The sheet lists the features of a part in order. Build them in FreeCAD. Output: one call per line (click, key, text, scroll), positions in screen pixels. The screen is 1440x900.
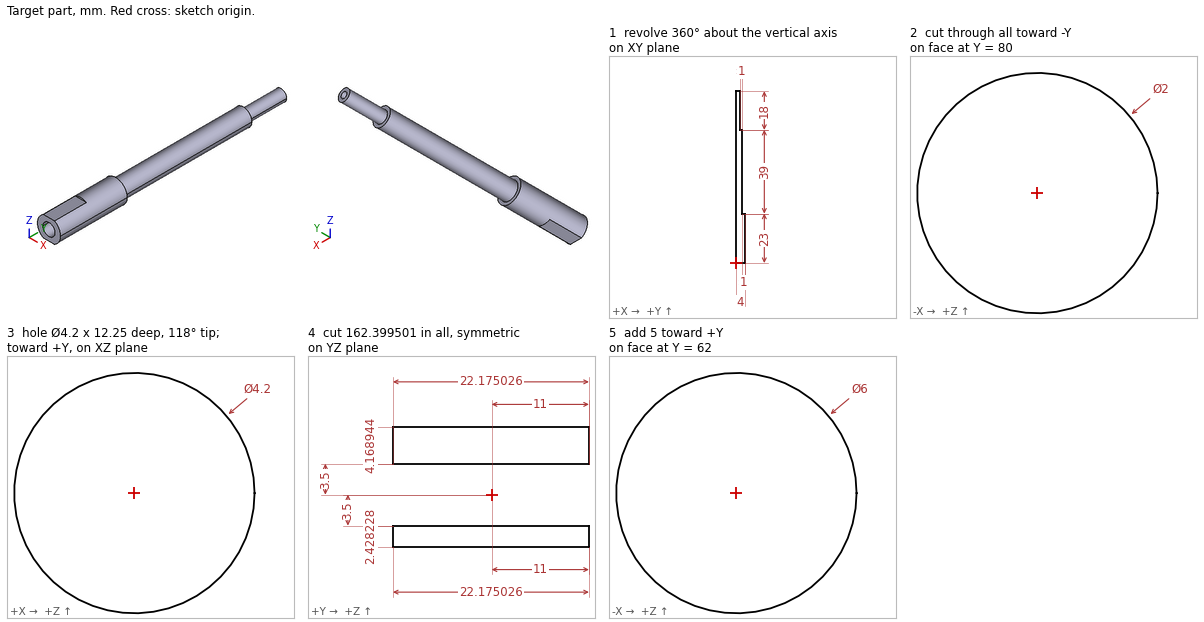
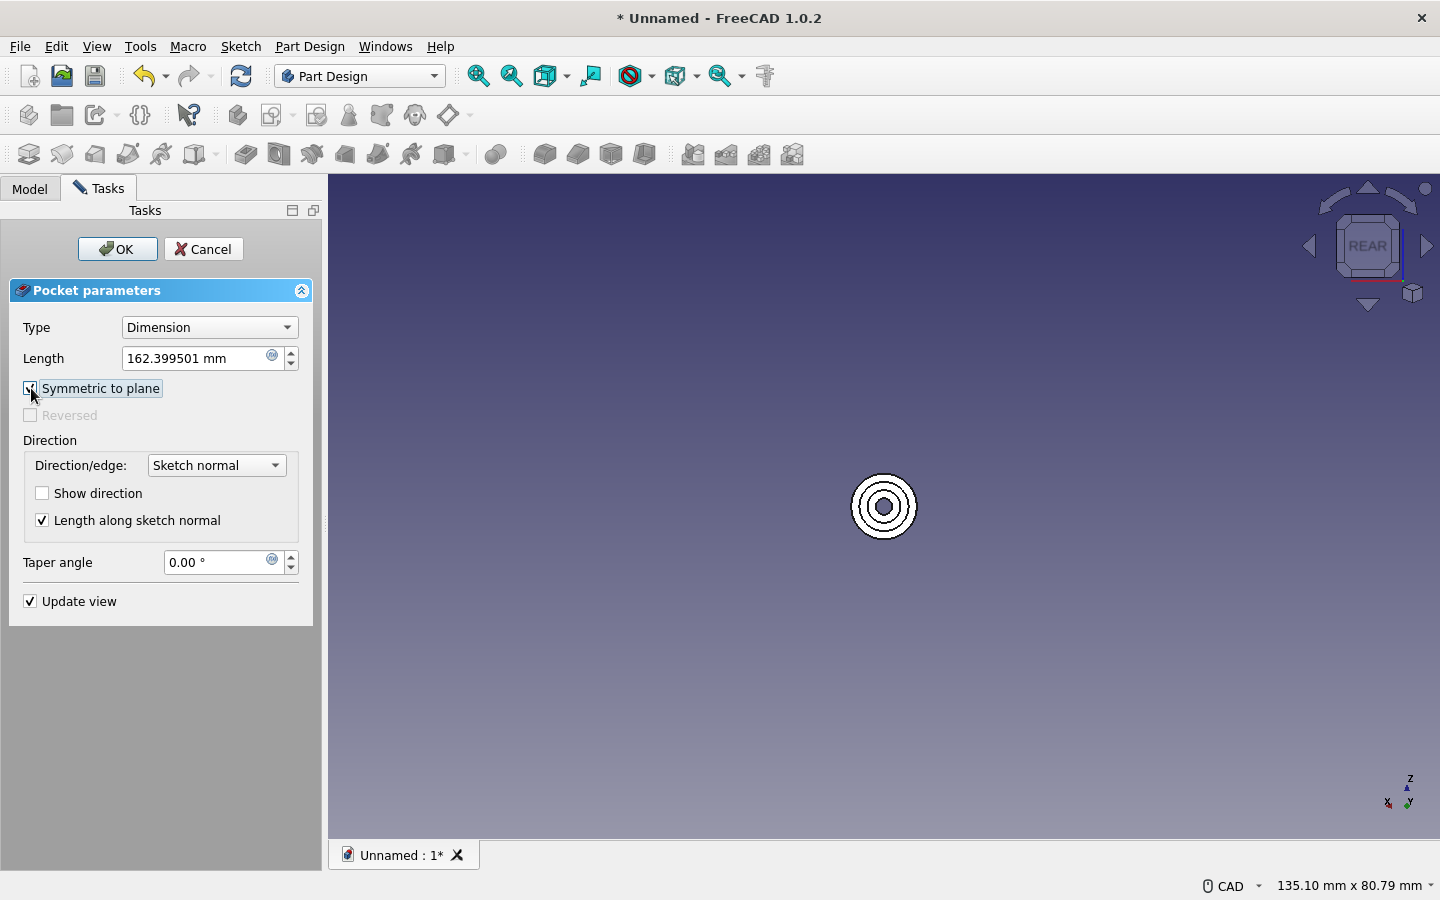
click(118, 249)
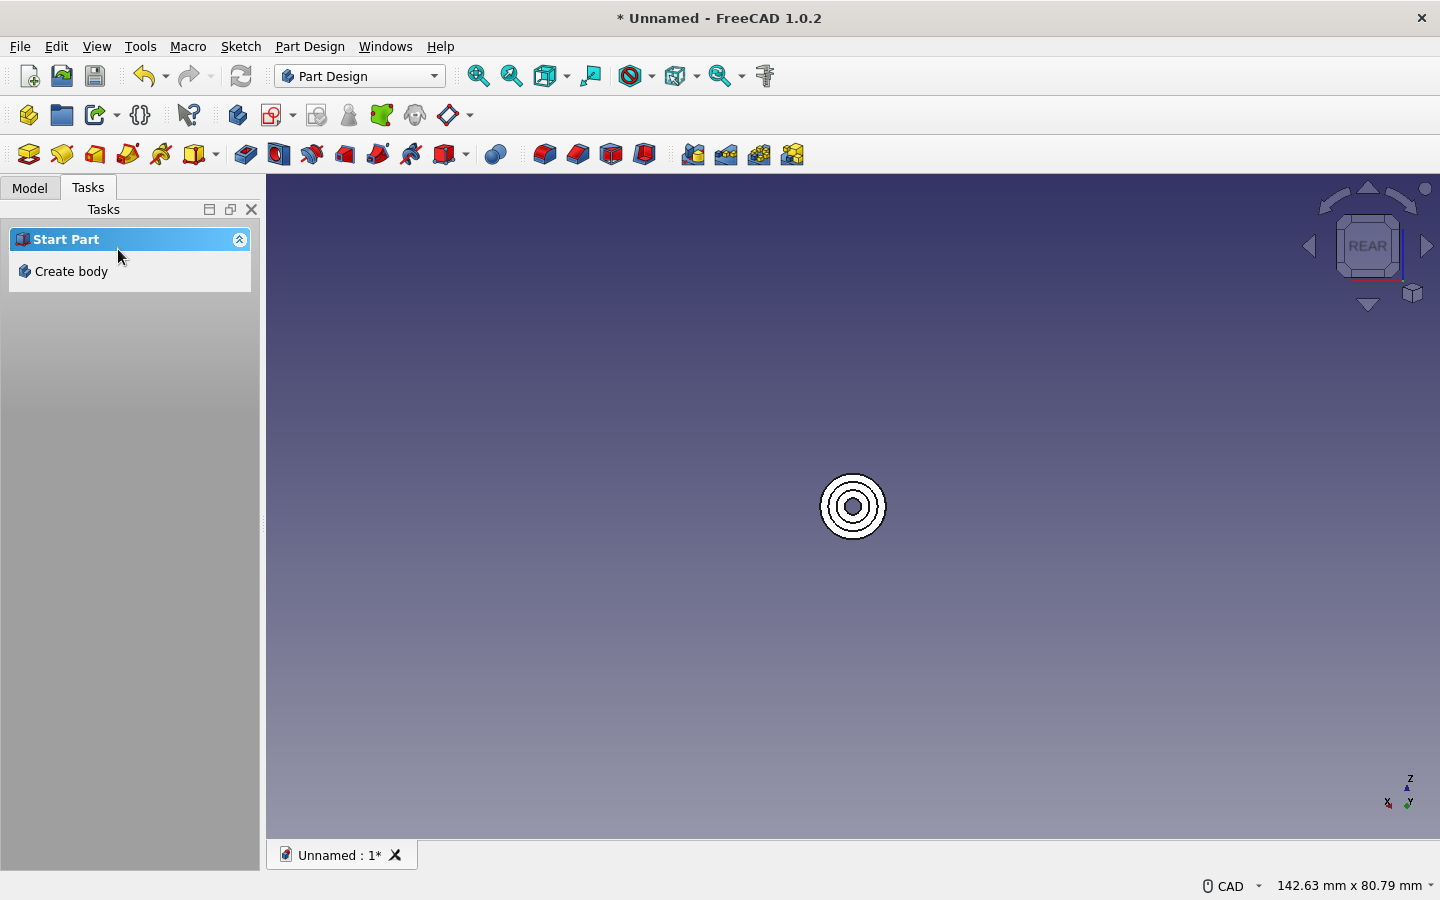
key(v)
key(f)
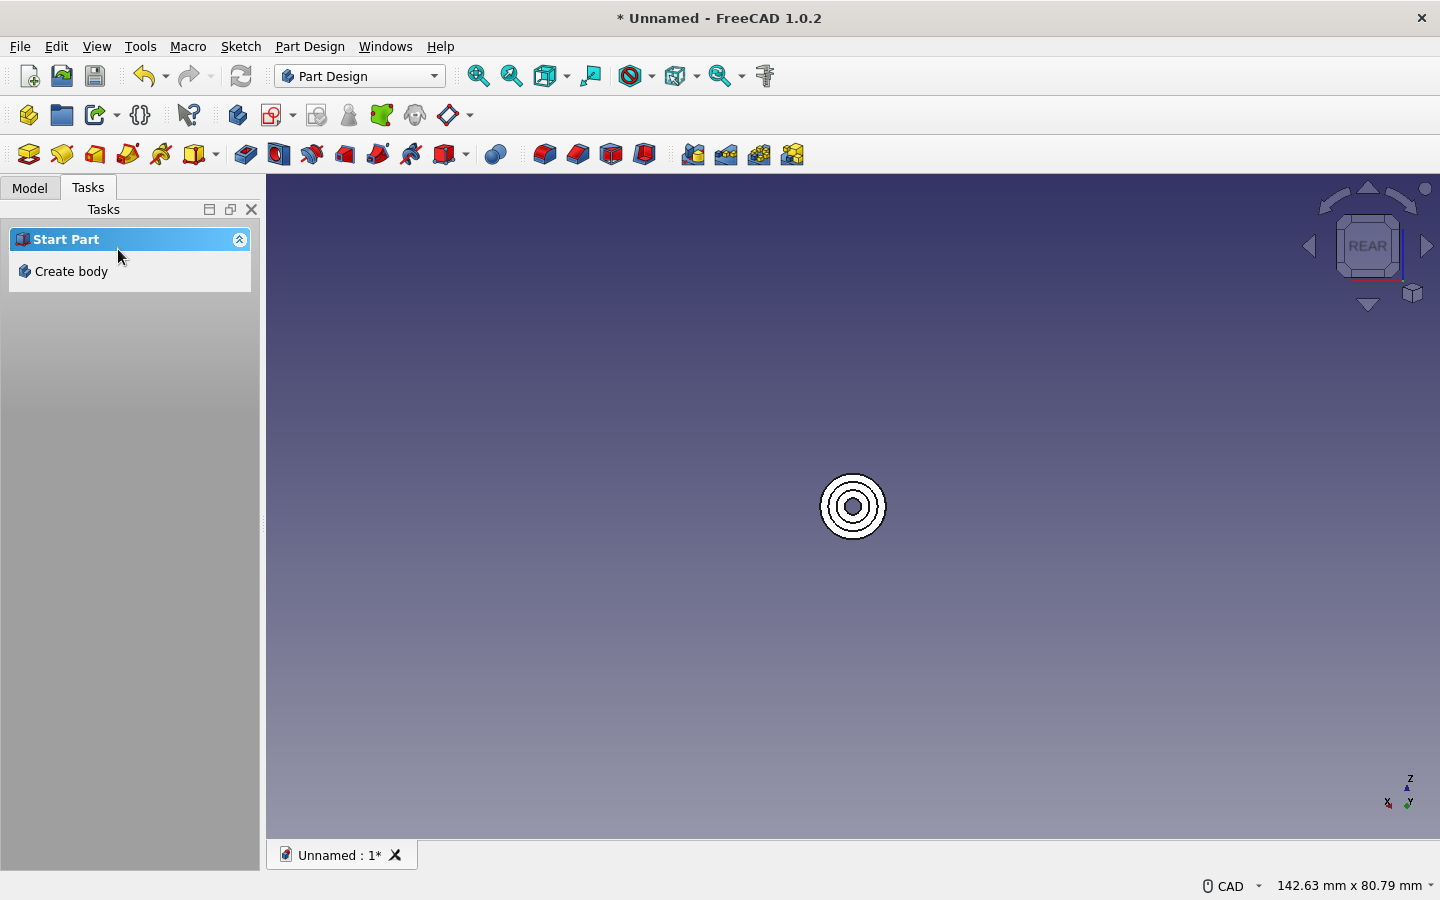
scroll(832, 505, up, 7)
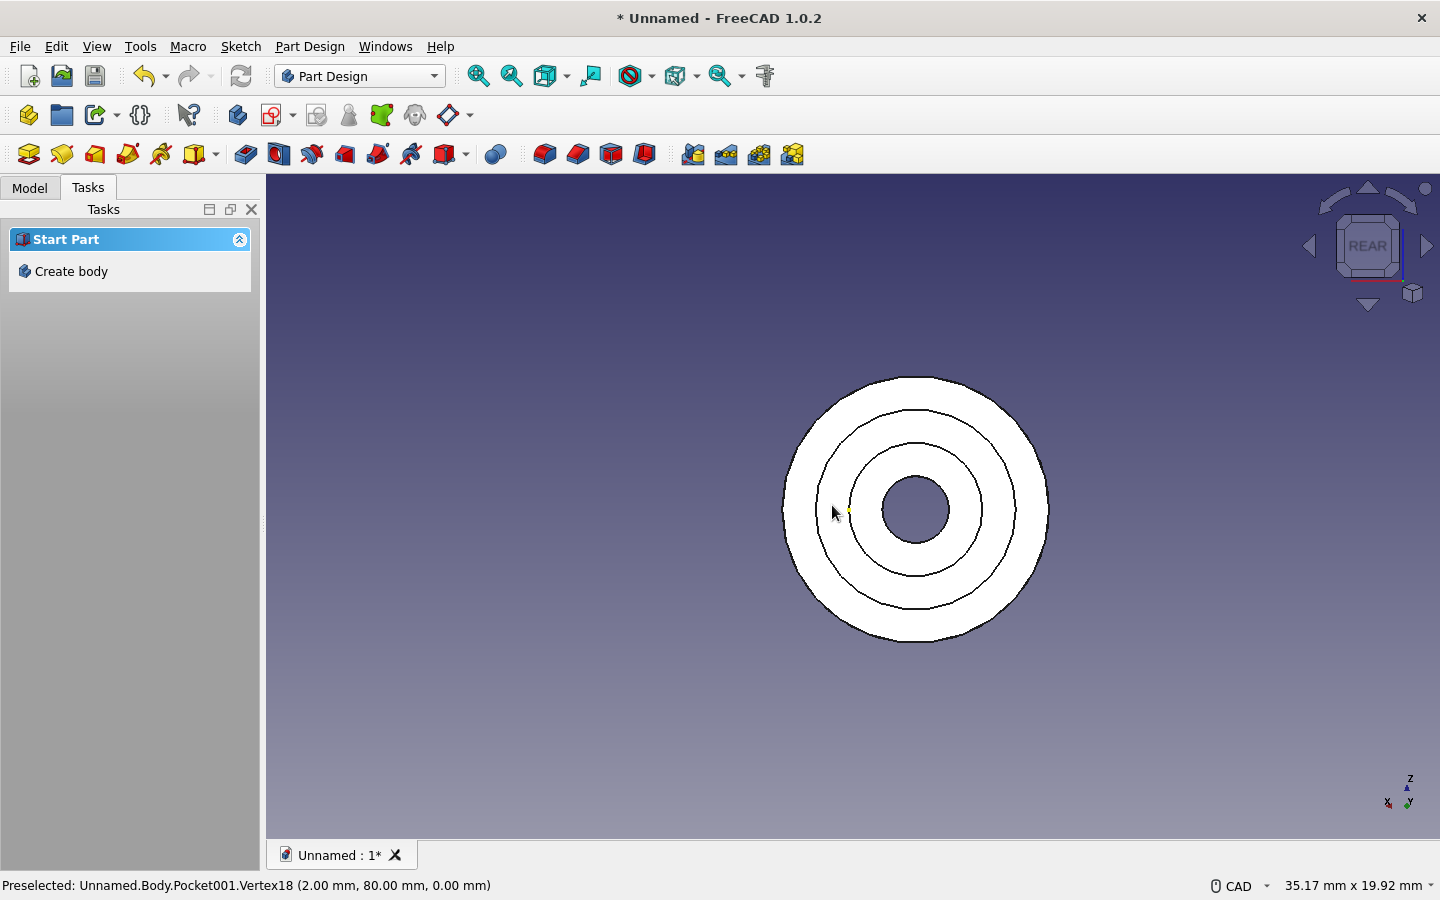
click(830, 509)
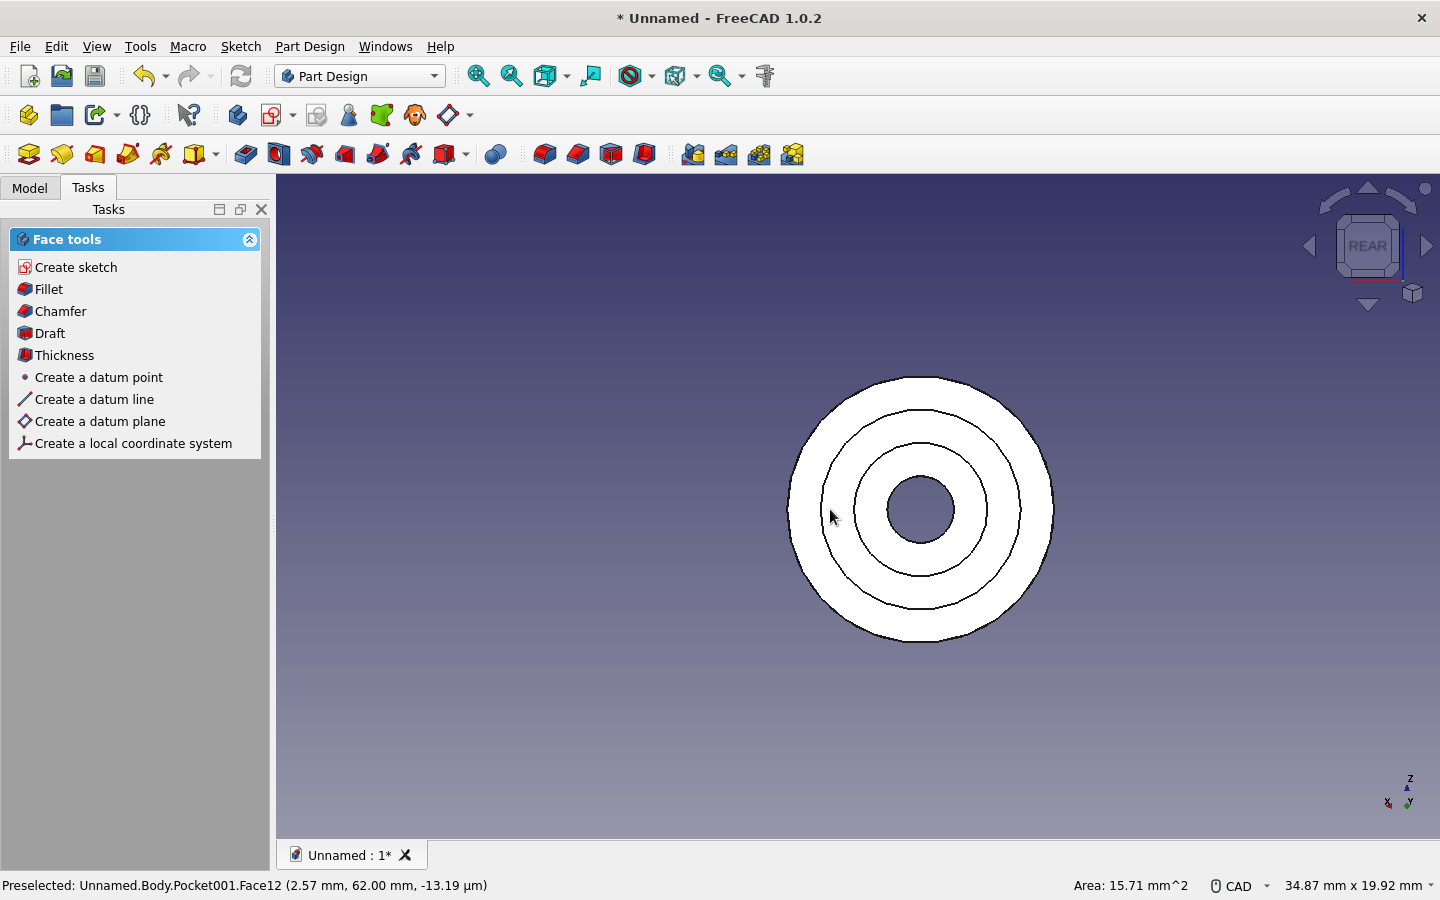
click(270, 116)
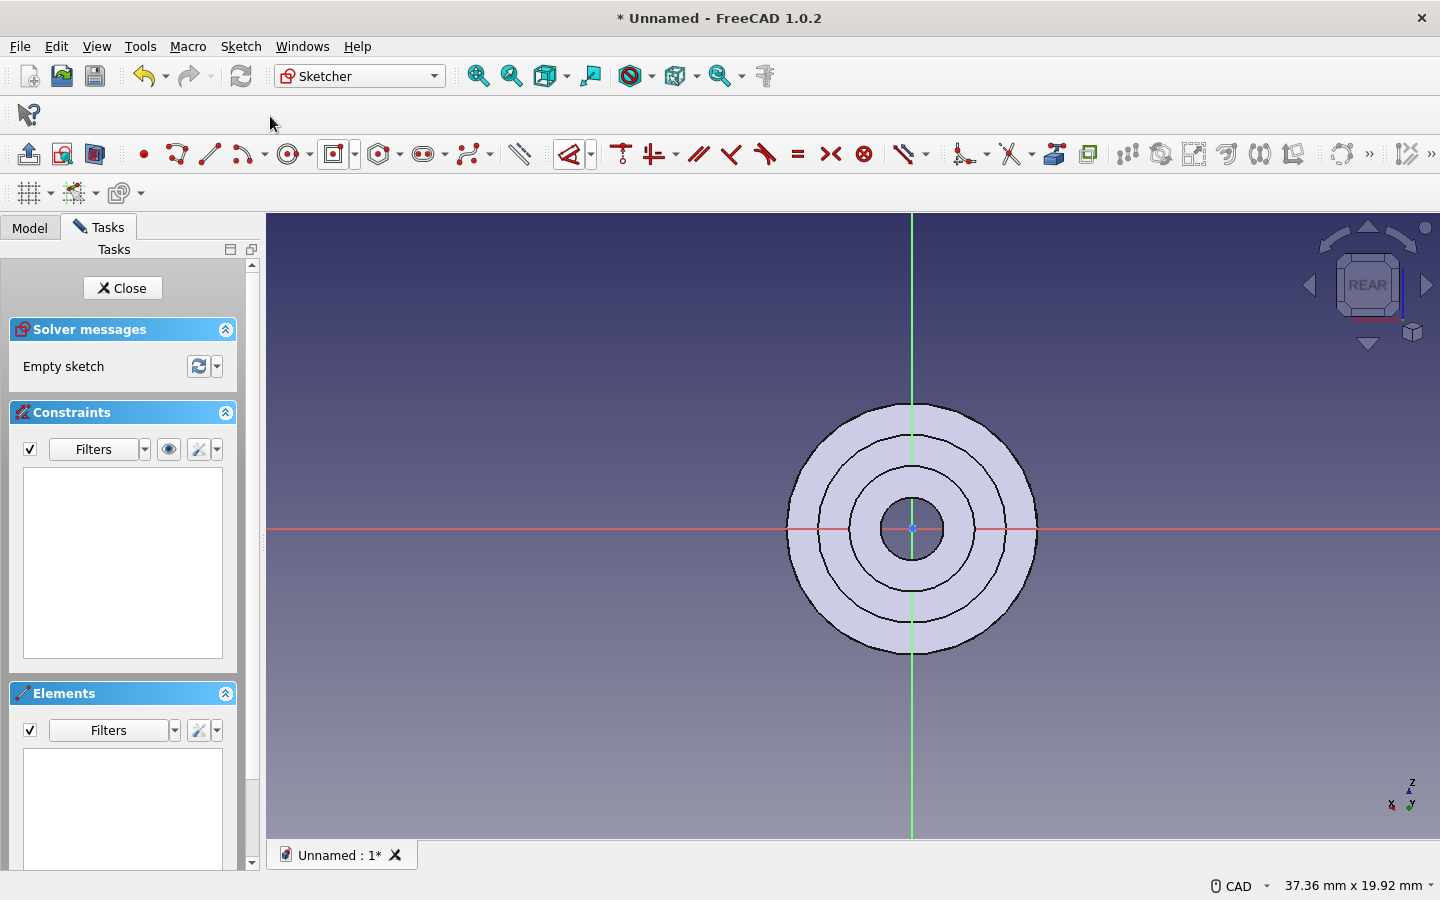
scroll(1016, 531, up, 4)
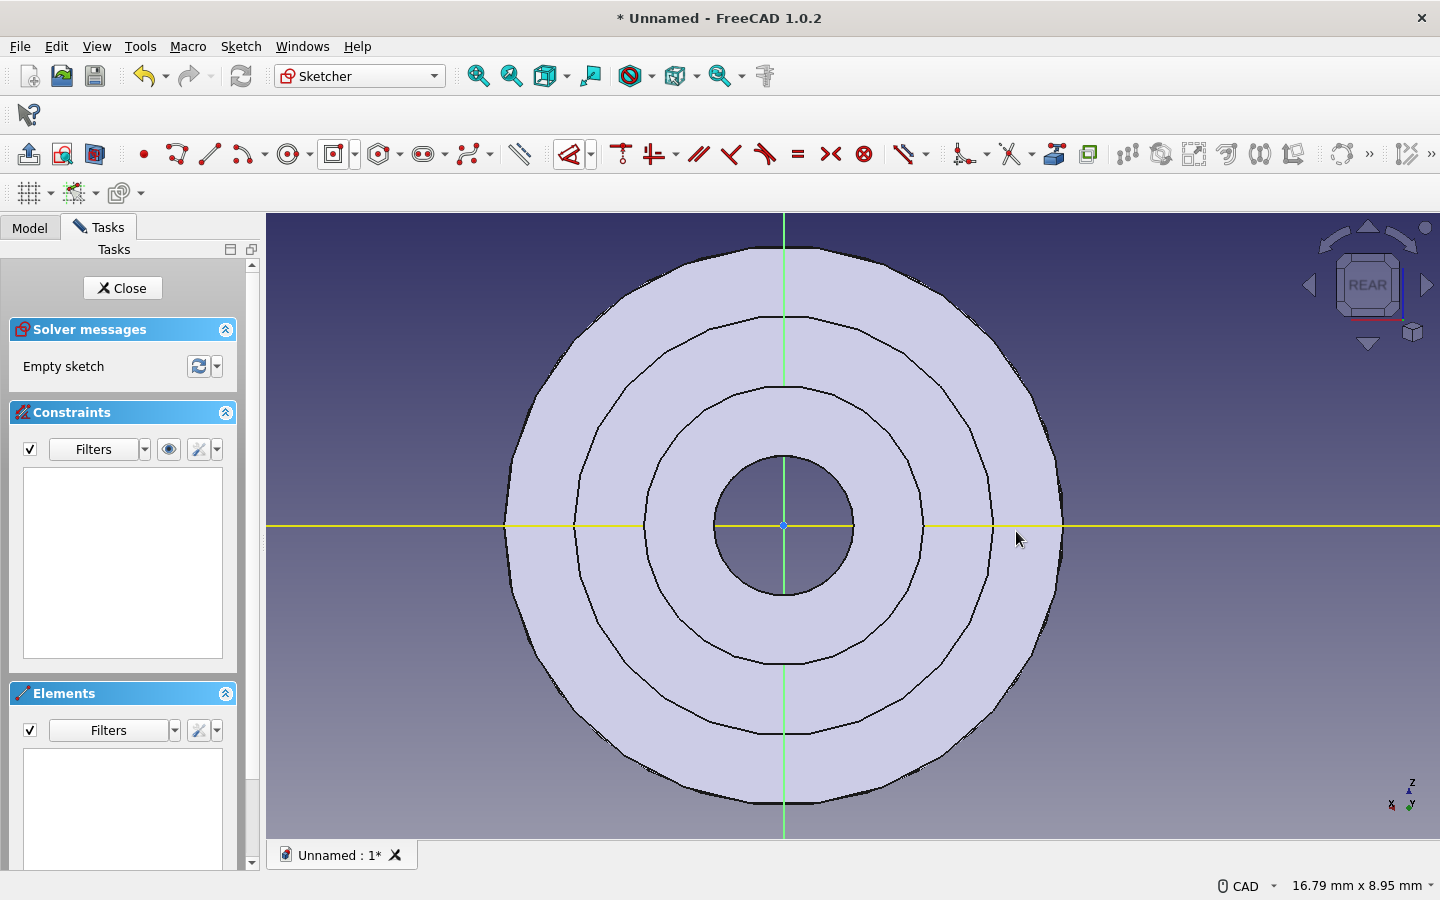
click(288, 154)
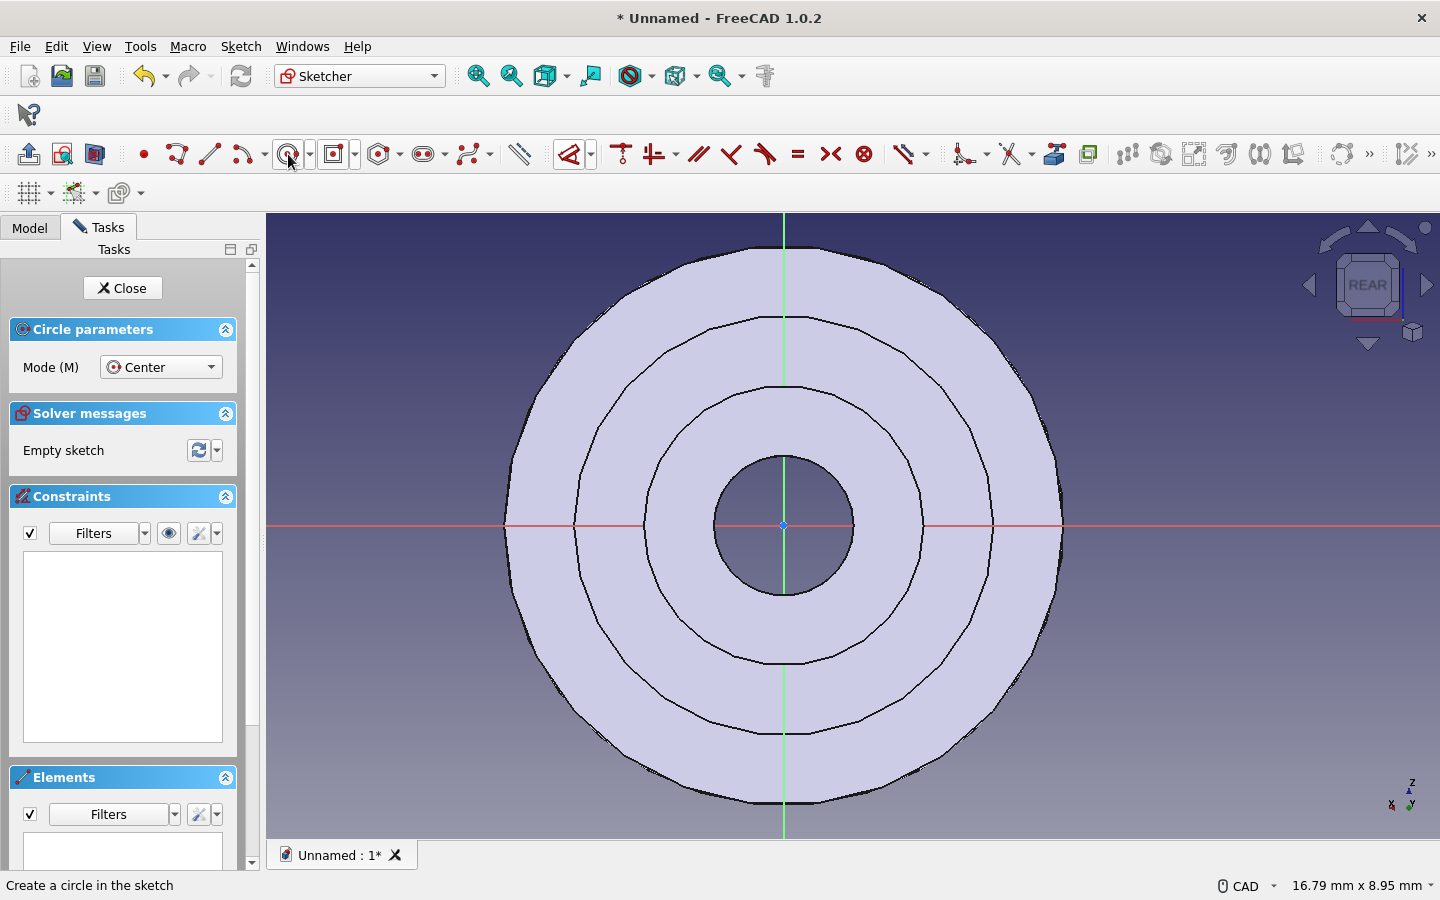
click(784, 526)
click(932, 377)
key(Escape)